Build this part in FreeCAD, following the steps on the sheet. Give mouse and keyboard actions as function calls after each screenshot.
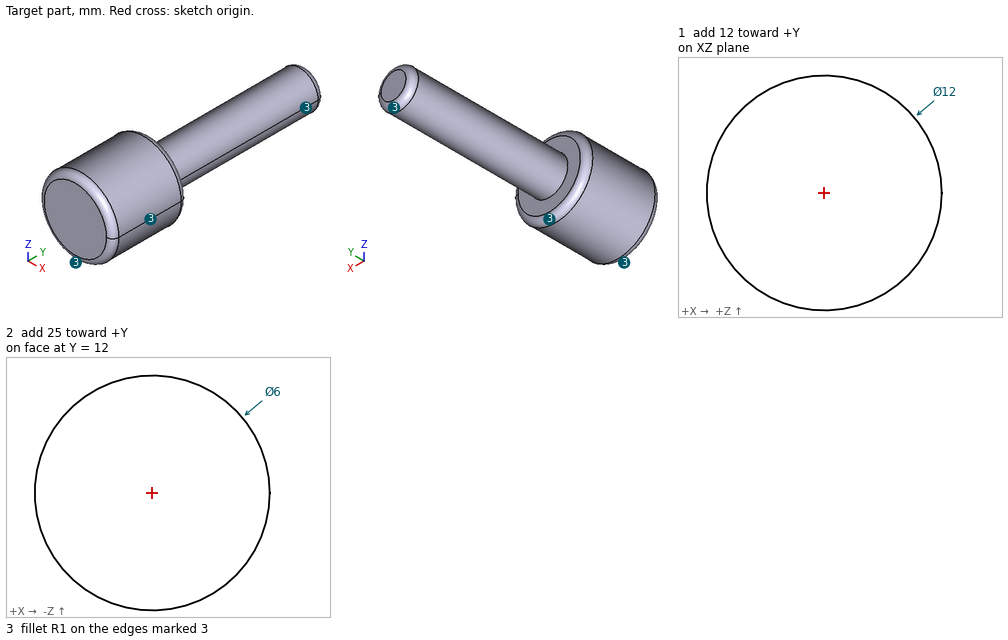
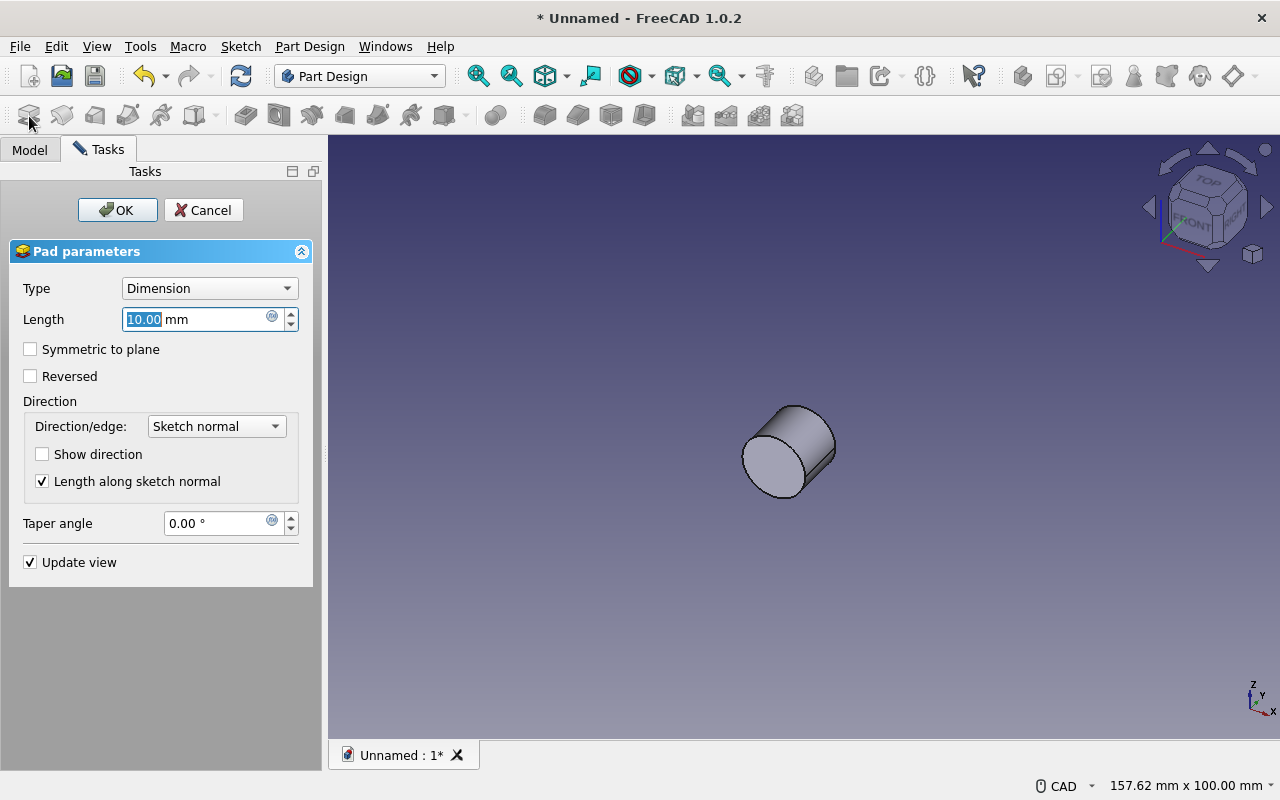
text(12)
key(Tab)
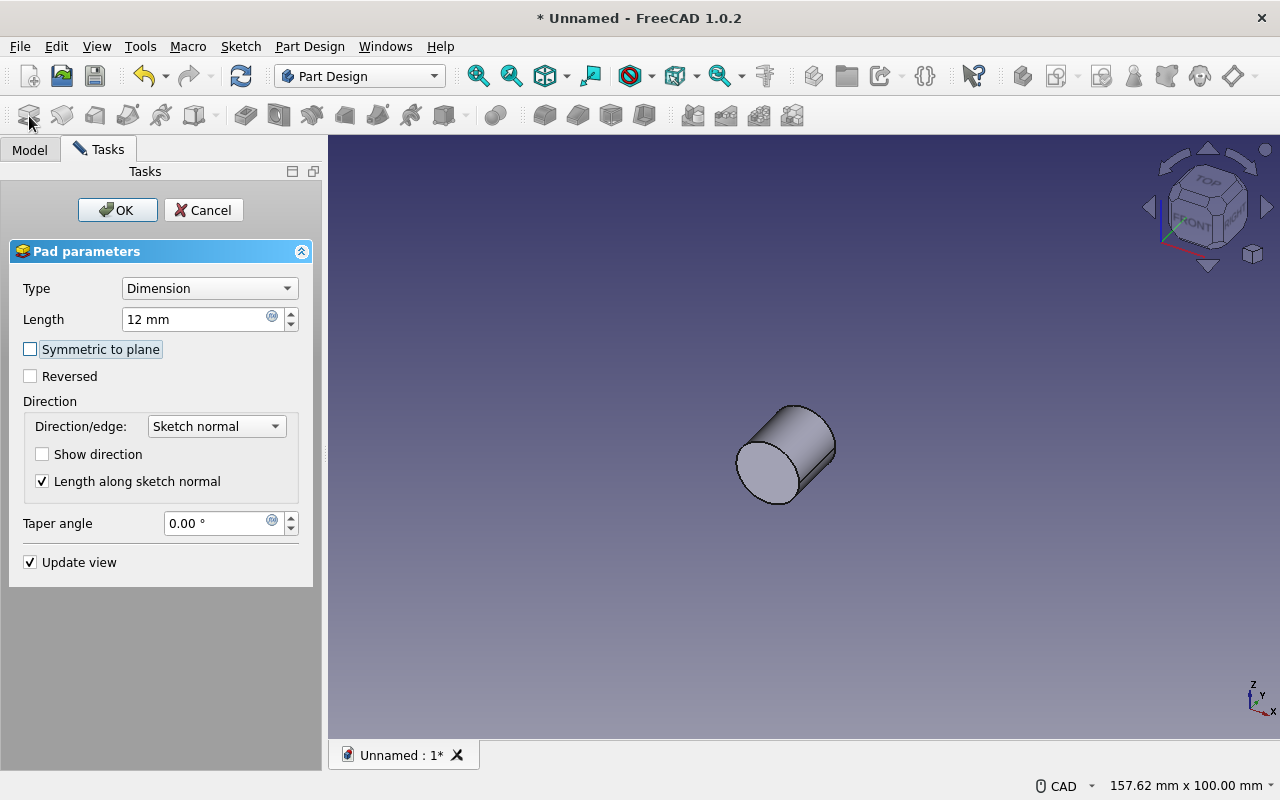
click(31, 376)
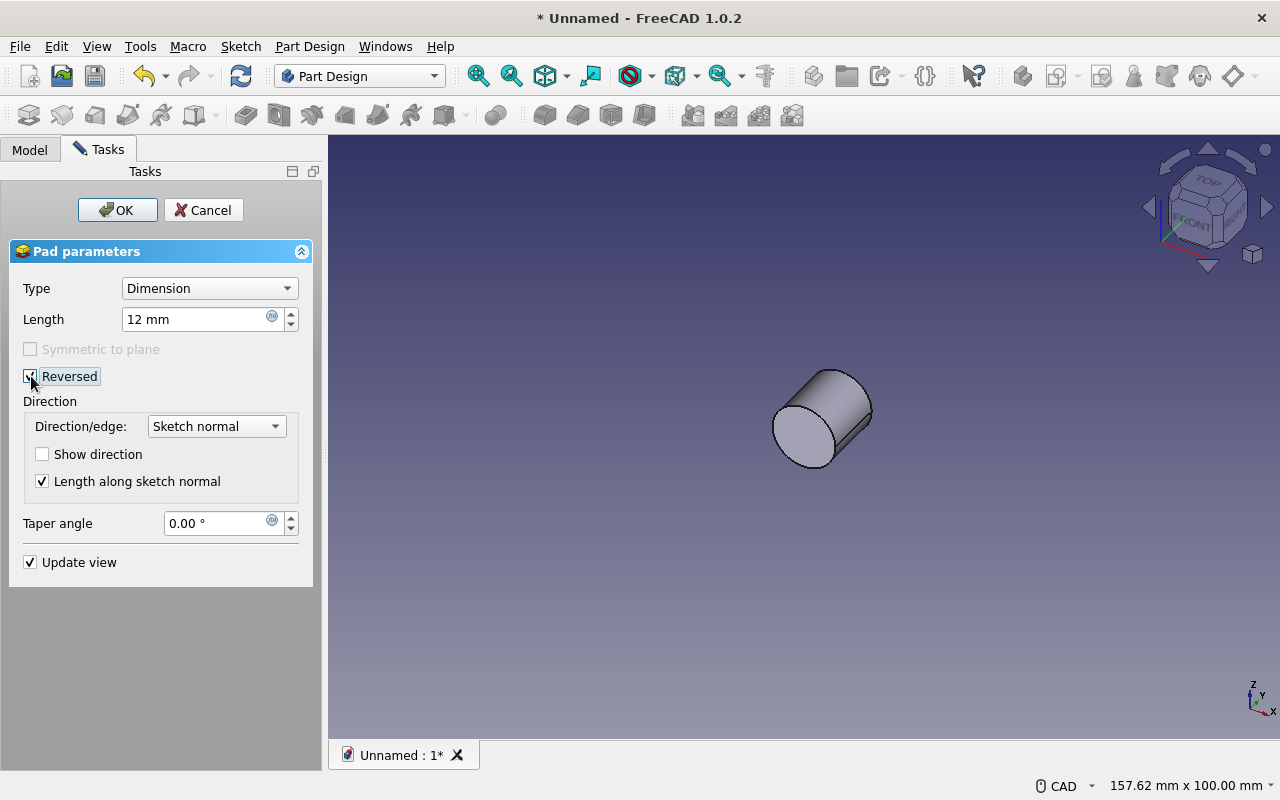
click(118, 210)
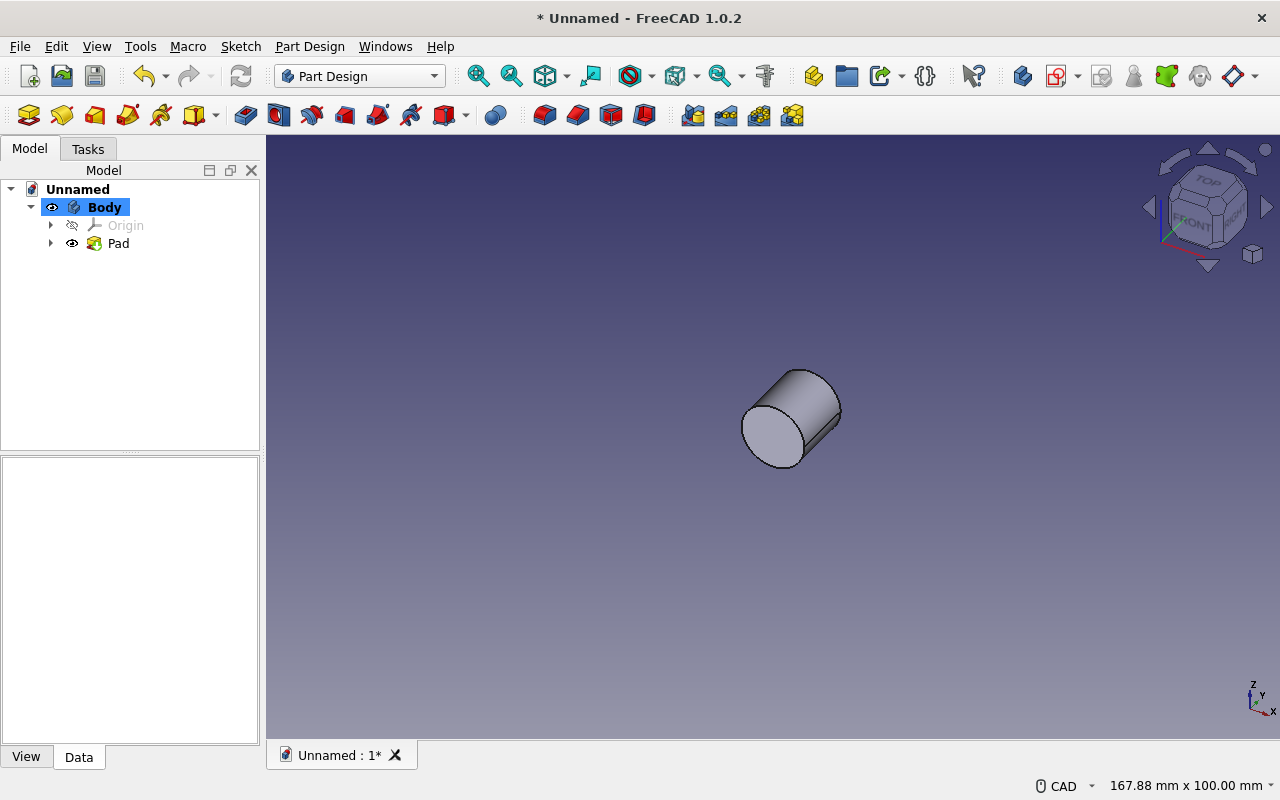
click(479, 76)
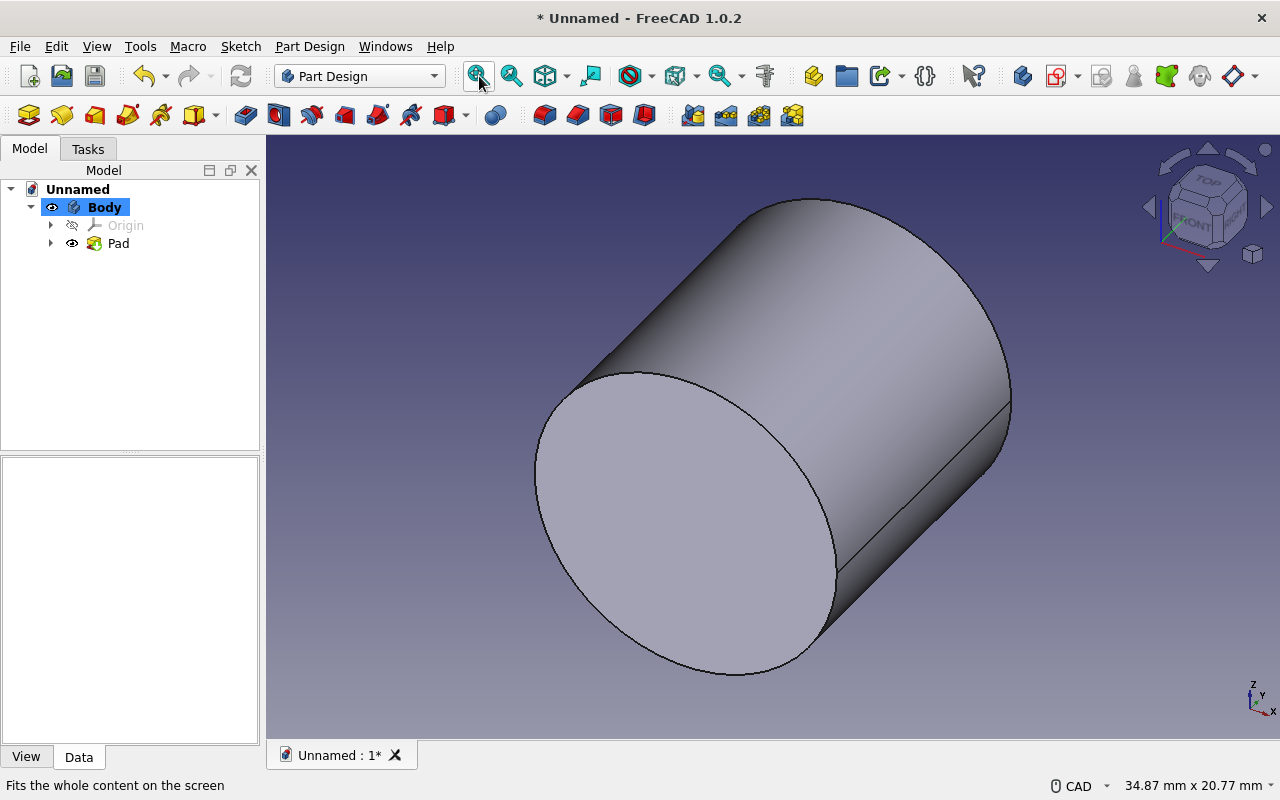
key(4)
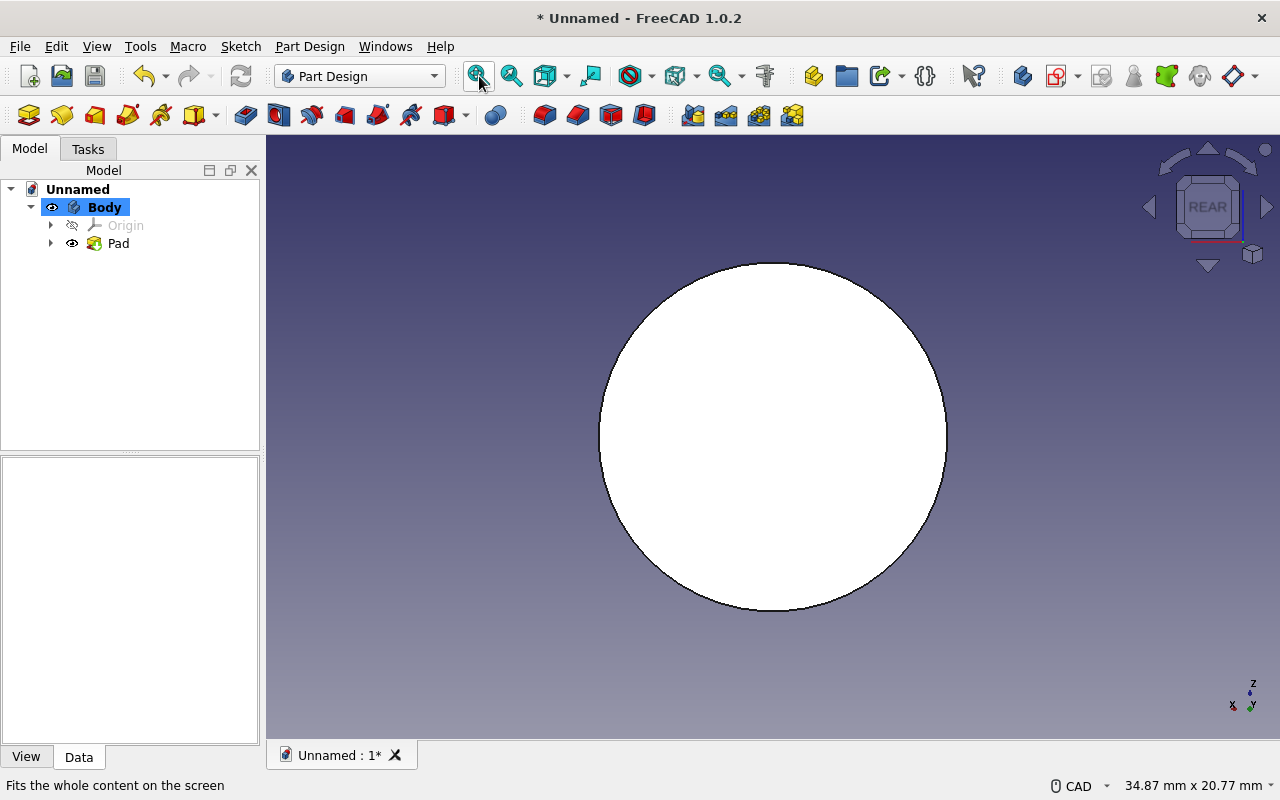
click(773, 436)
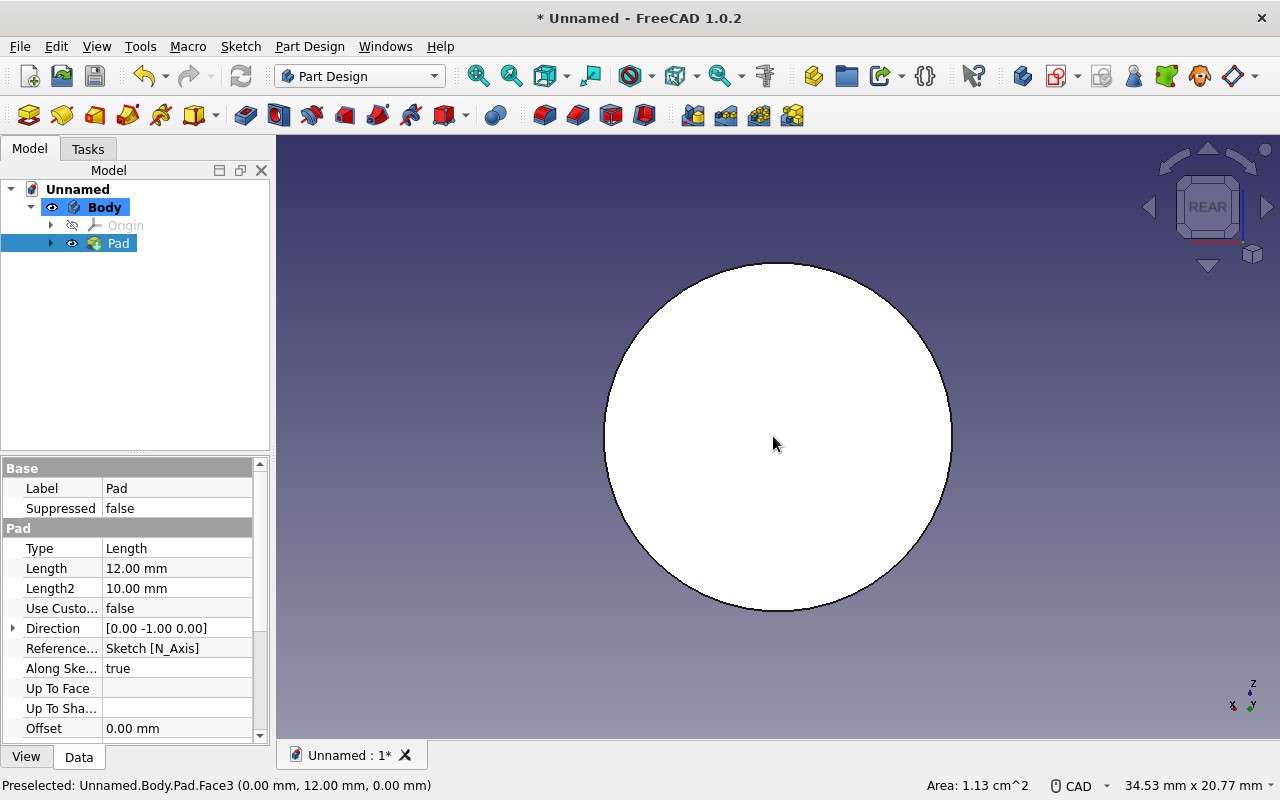
click(1056, 76)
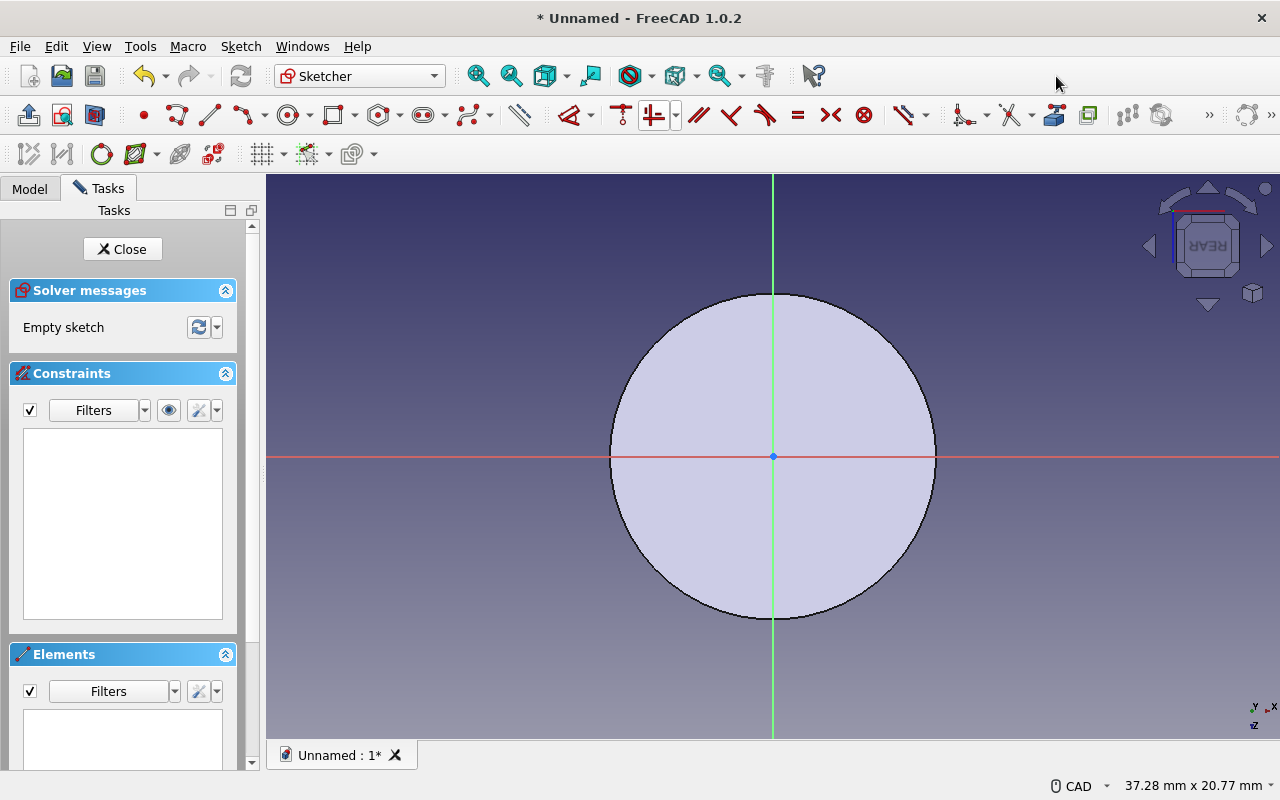
scroll(829, 456, up, 4)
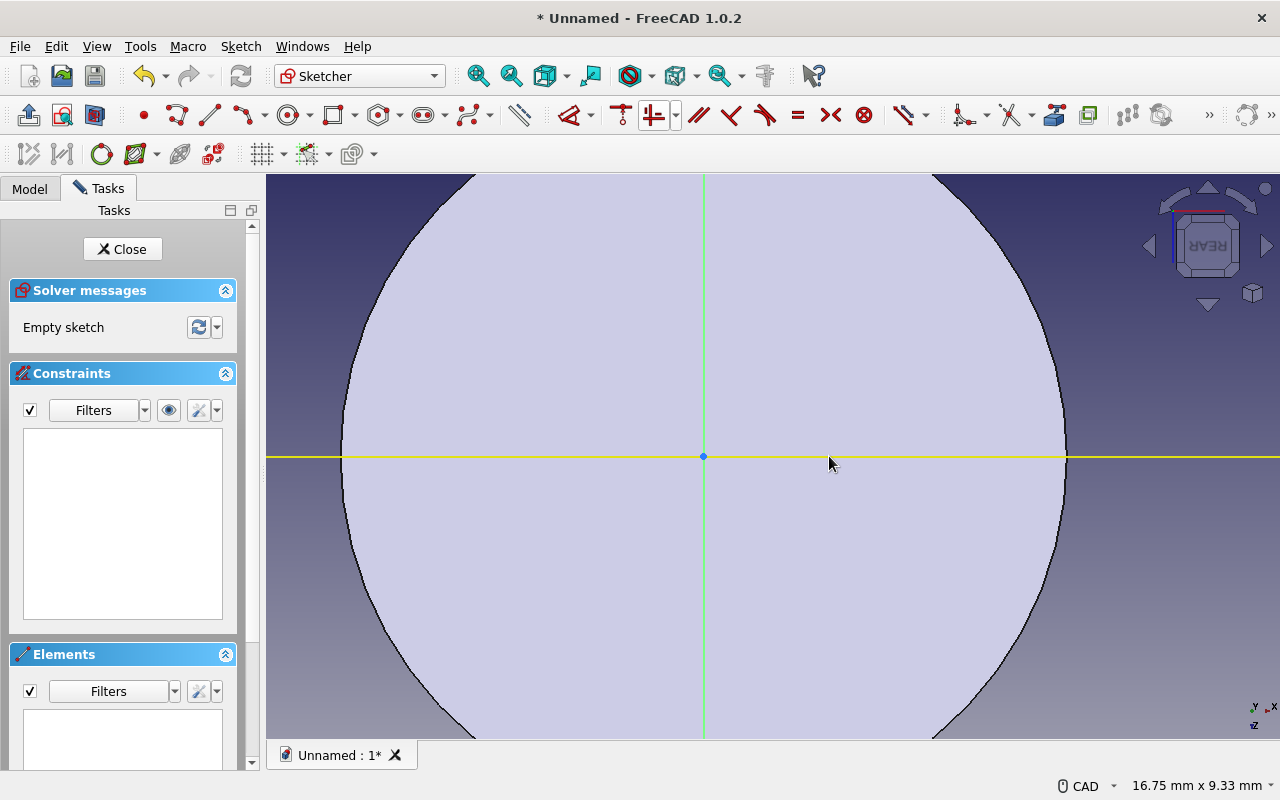
click(288, 116)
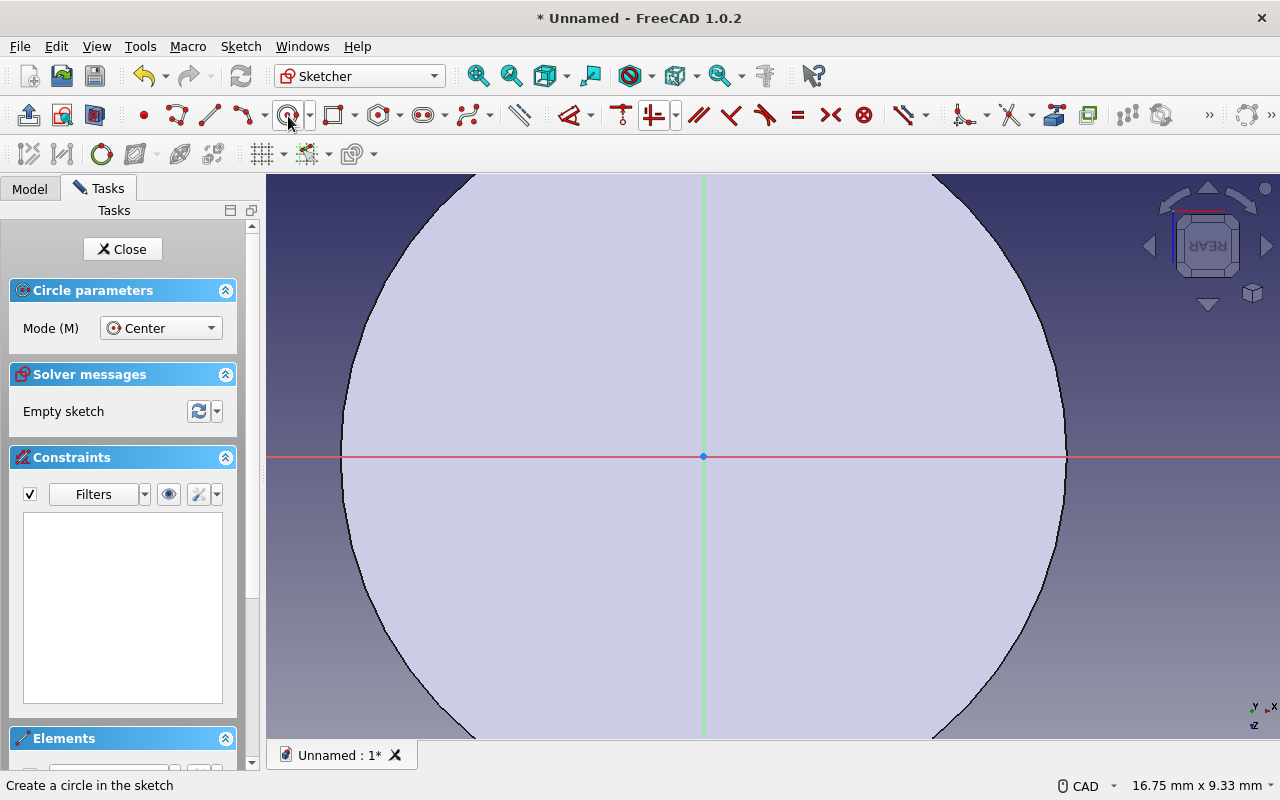
click(704, 456)
move(832, 328)